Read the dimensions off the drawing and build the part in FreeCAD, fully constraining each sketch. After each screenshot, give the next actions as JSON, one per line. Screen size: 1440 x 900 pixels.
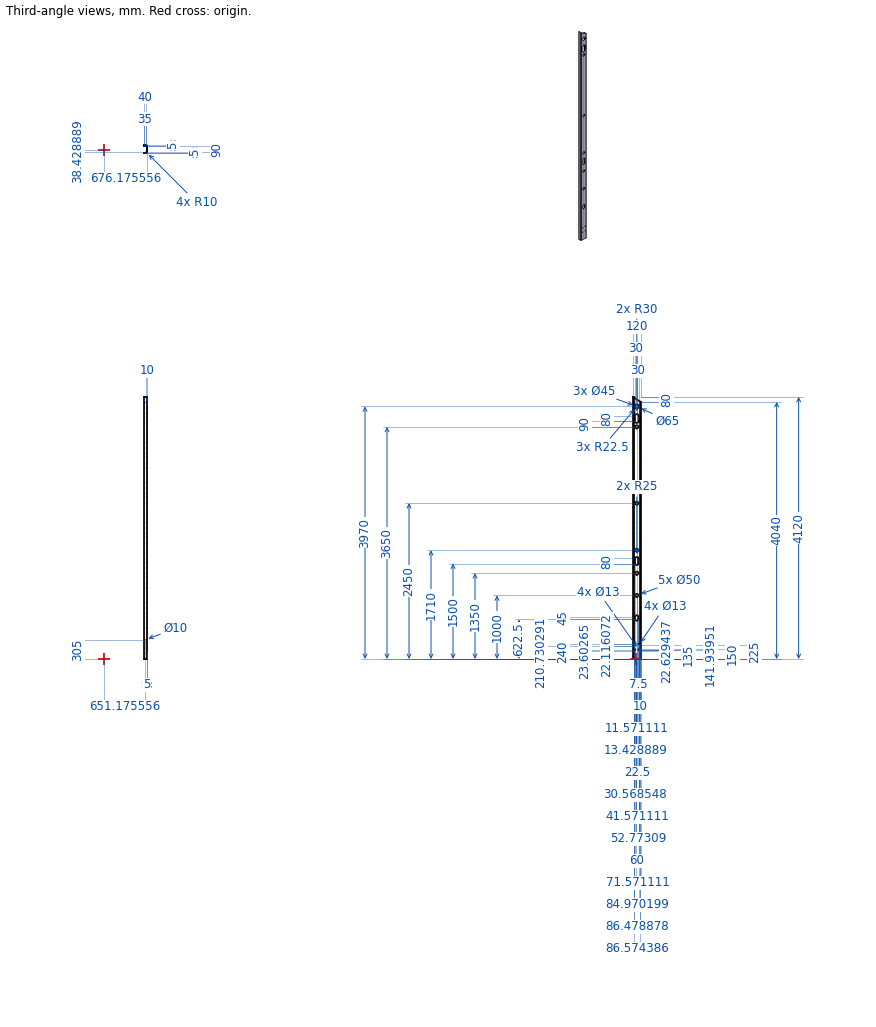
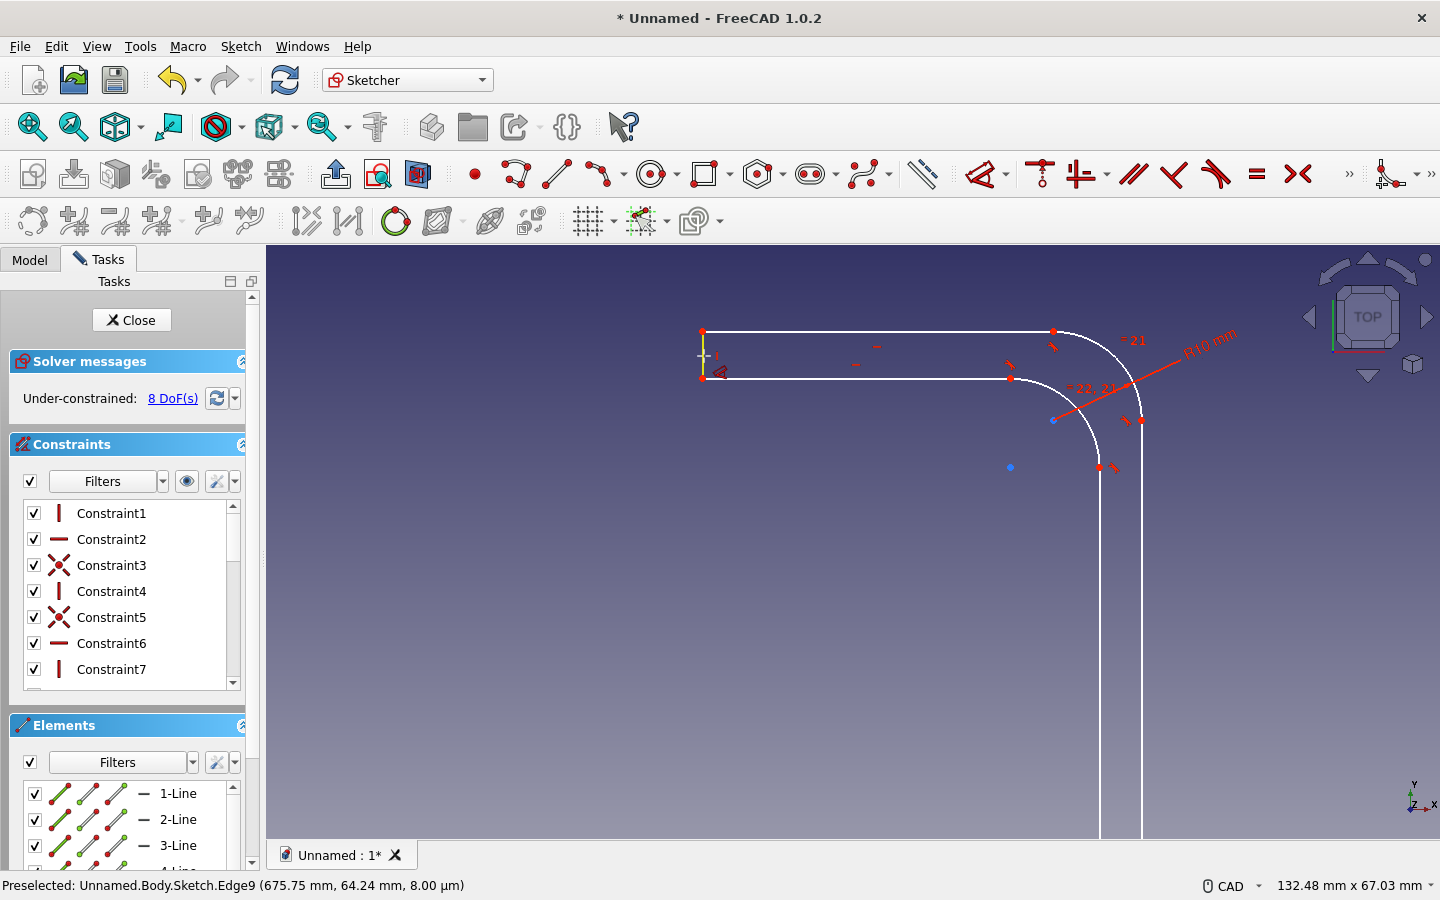
{"action": "left_click", "coordinate": [703, 355]}
{"action": "left_click", "coordinate": [669, 355]}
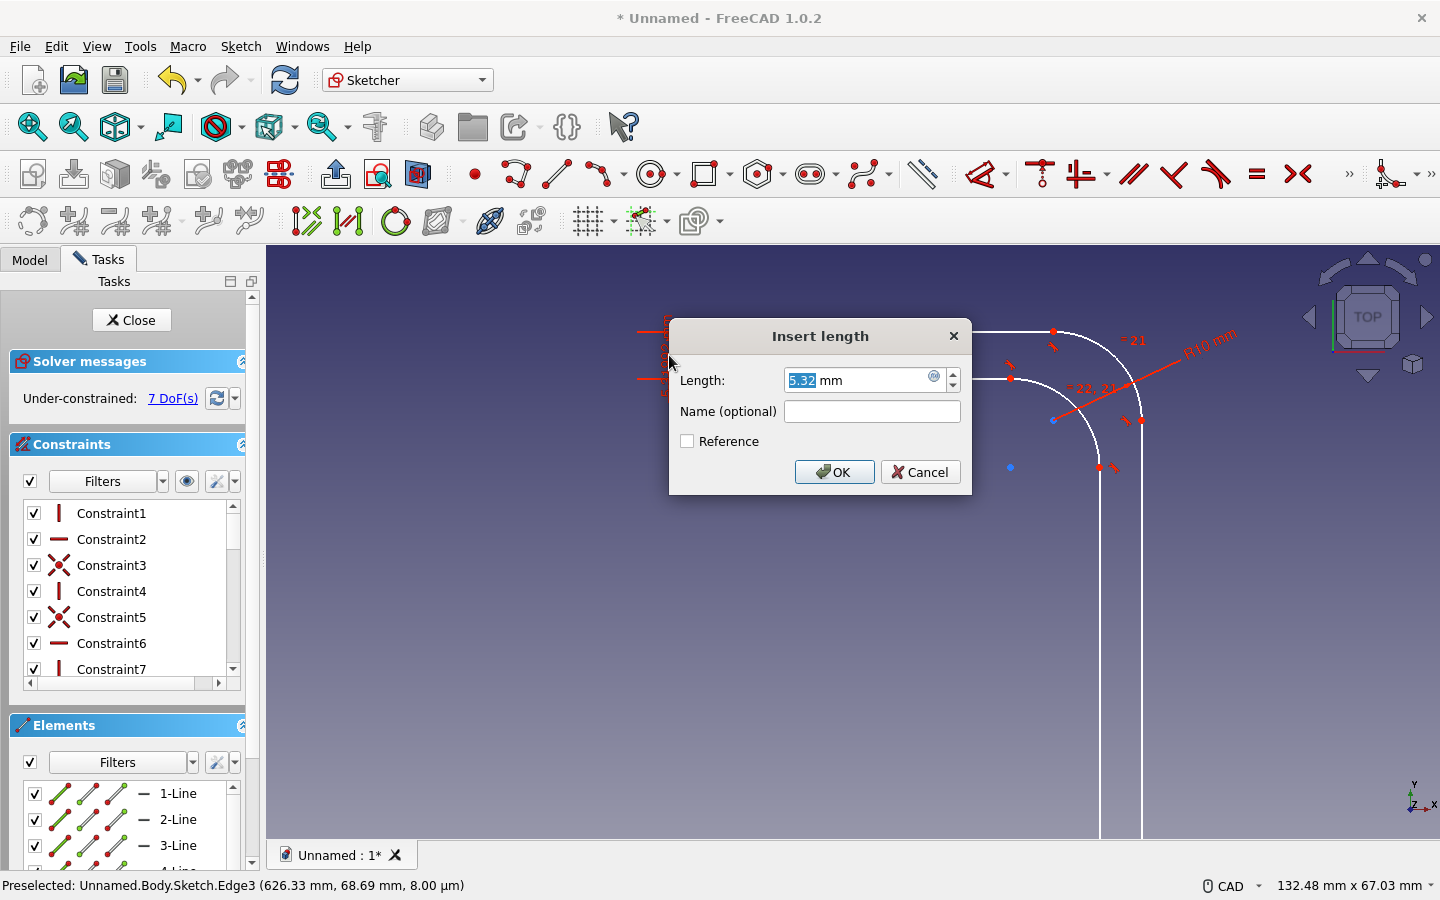
{"action": "type", "text": "5"}
{"action": "key", "text": "Return"}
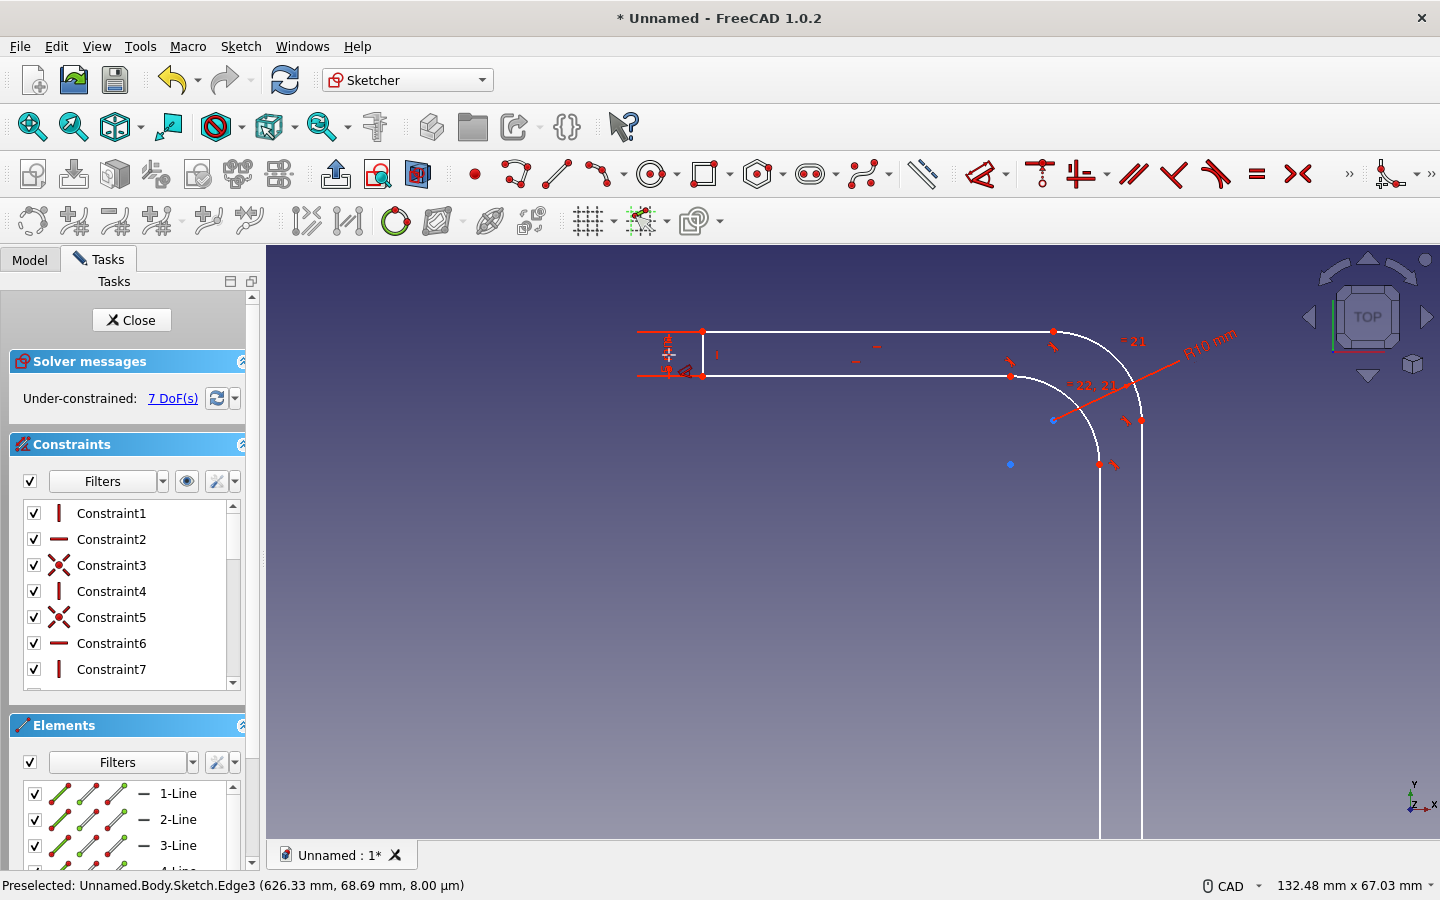
{"action": "scroll", "coordinate": [704, 356], "scroll_direction": "down", "scroll_amount": 5}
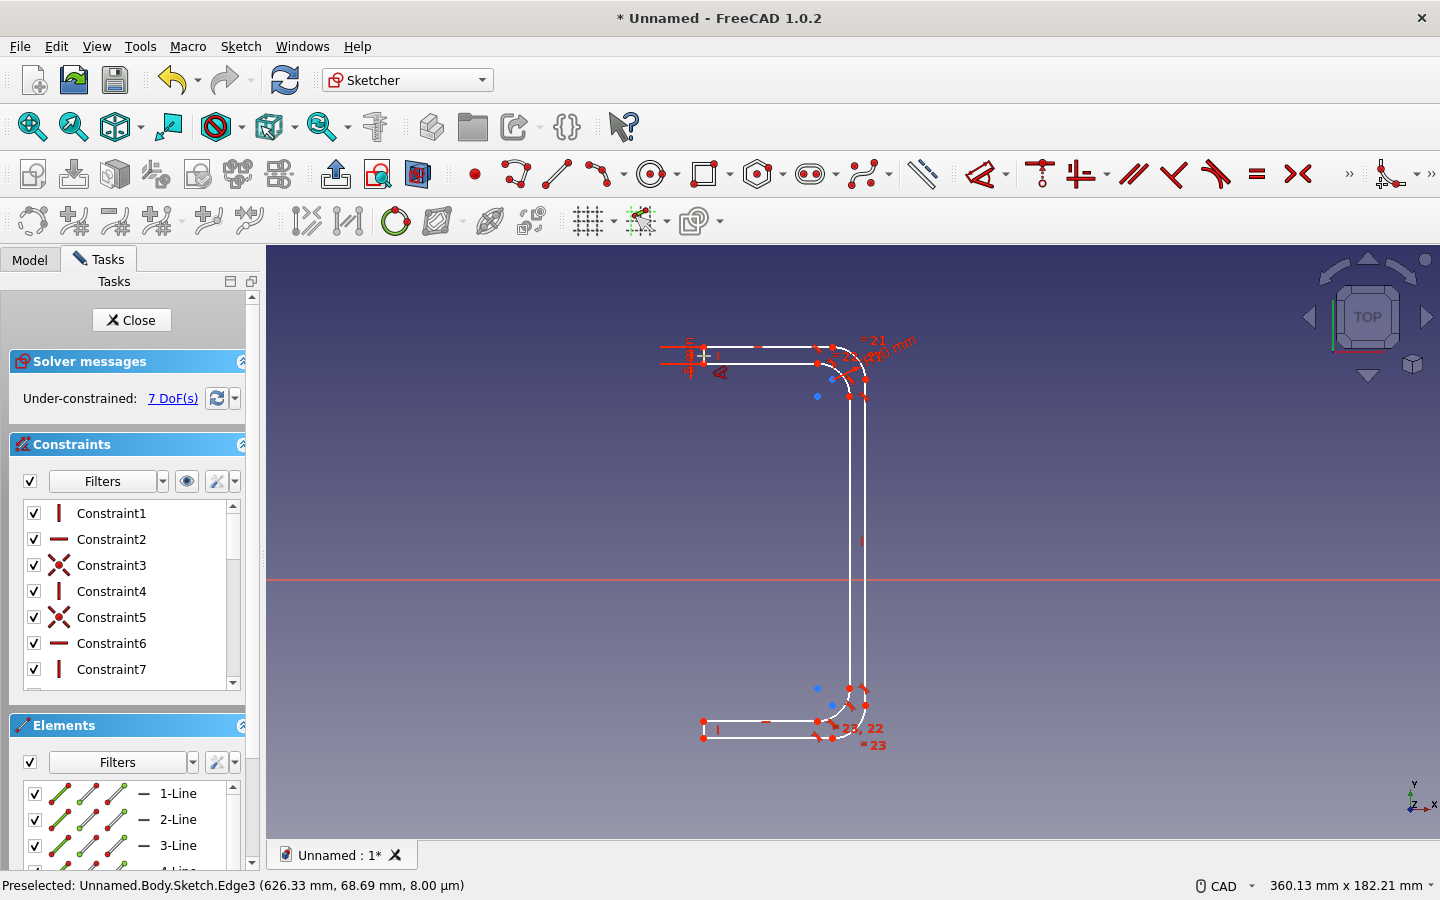
{"action": "scroll", "coordinate": [704, 726], "scroll_direction": "up", "scroll_amount": 5}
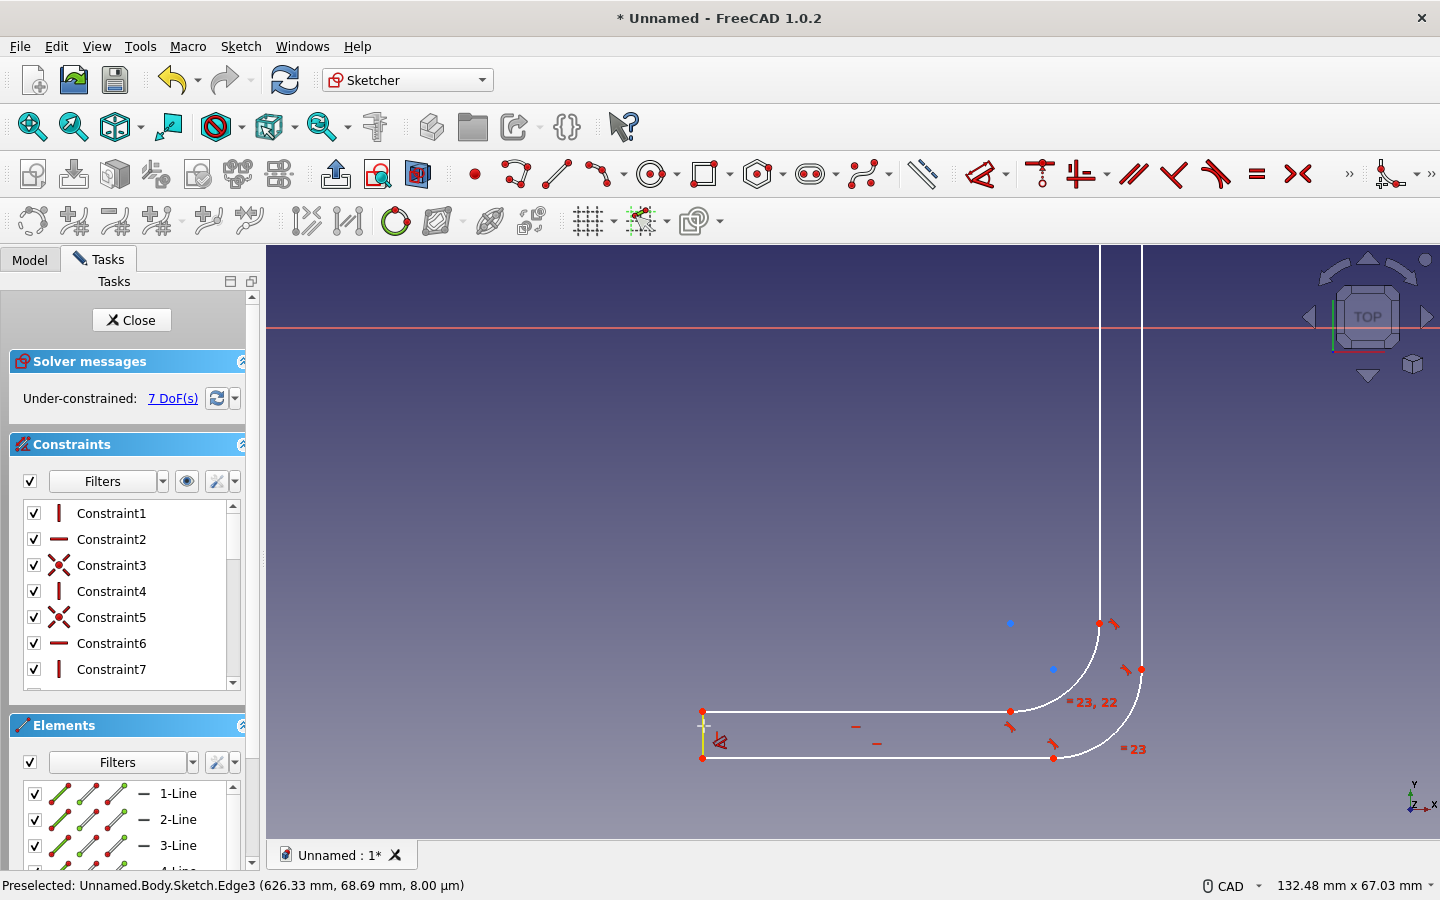
{"action": "left_click", "coordinate": [703, 726]}
{"action": "left_click", "coordinate": [669, 735]}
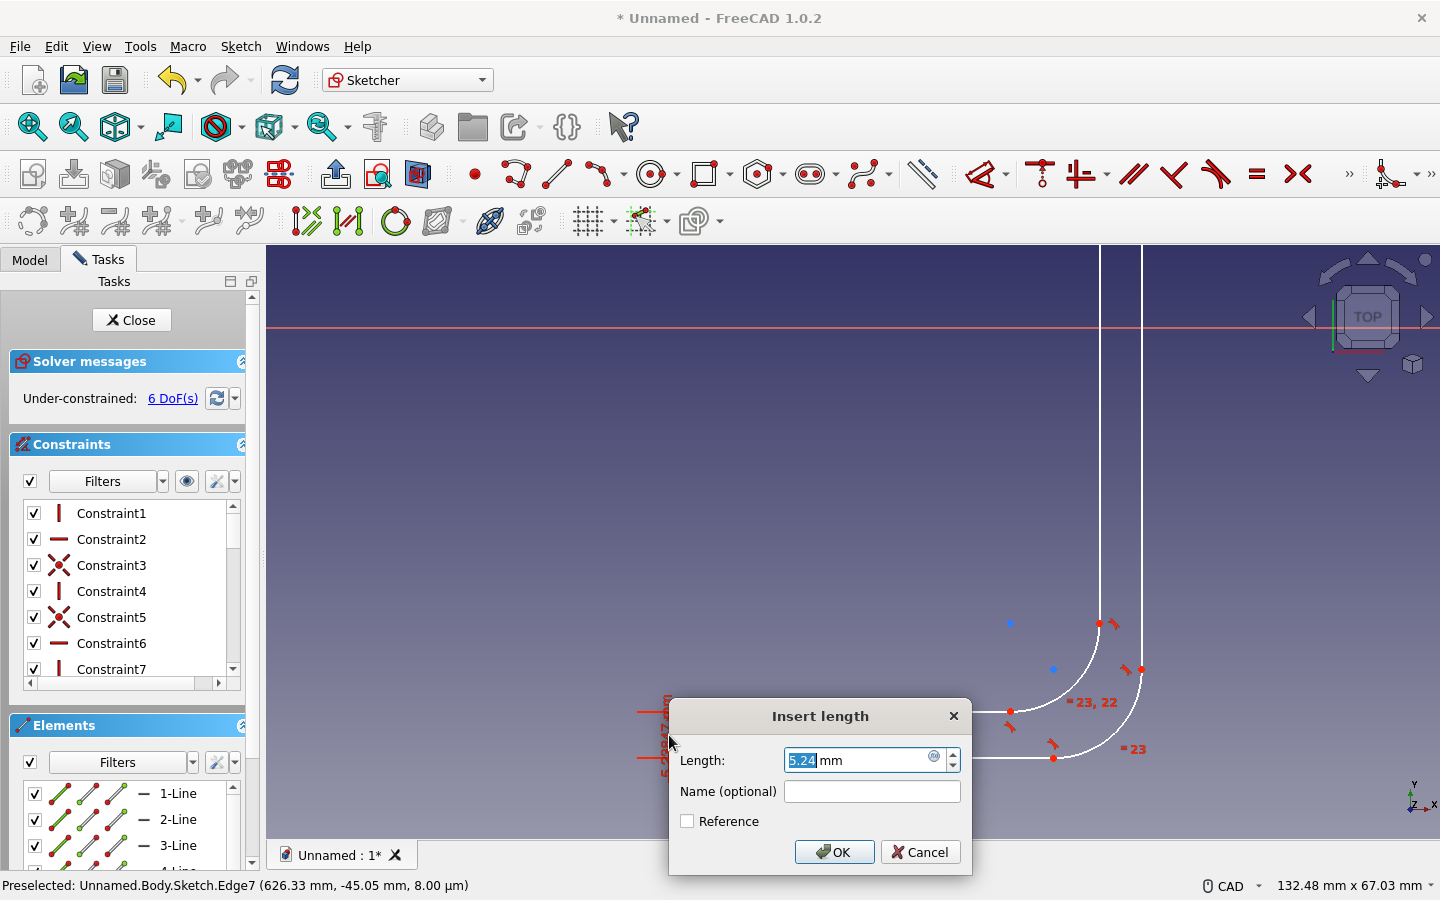
{"action": "type", "text": "5"}
{"action": "key", "text": "Return"}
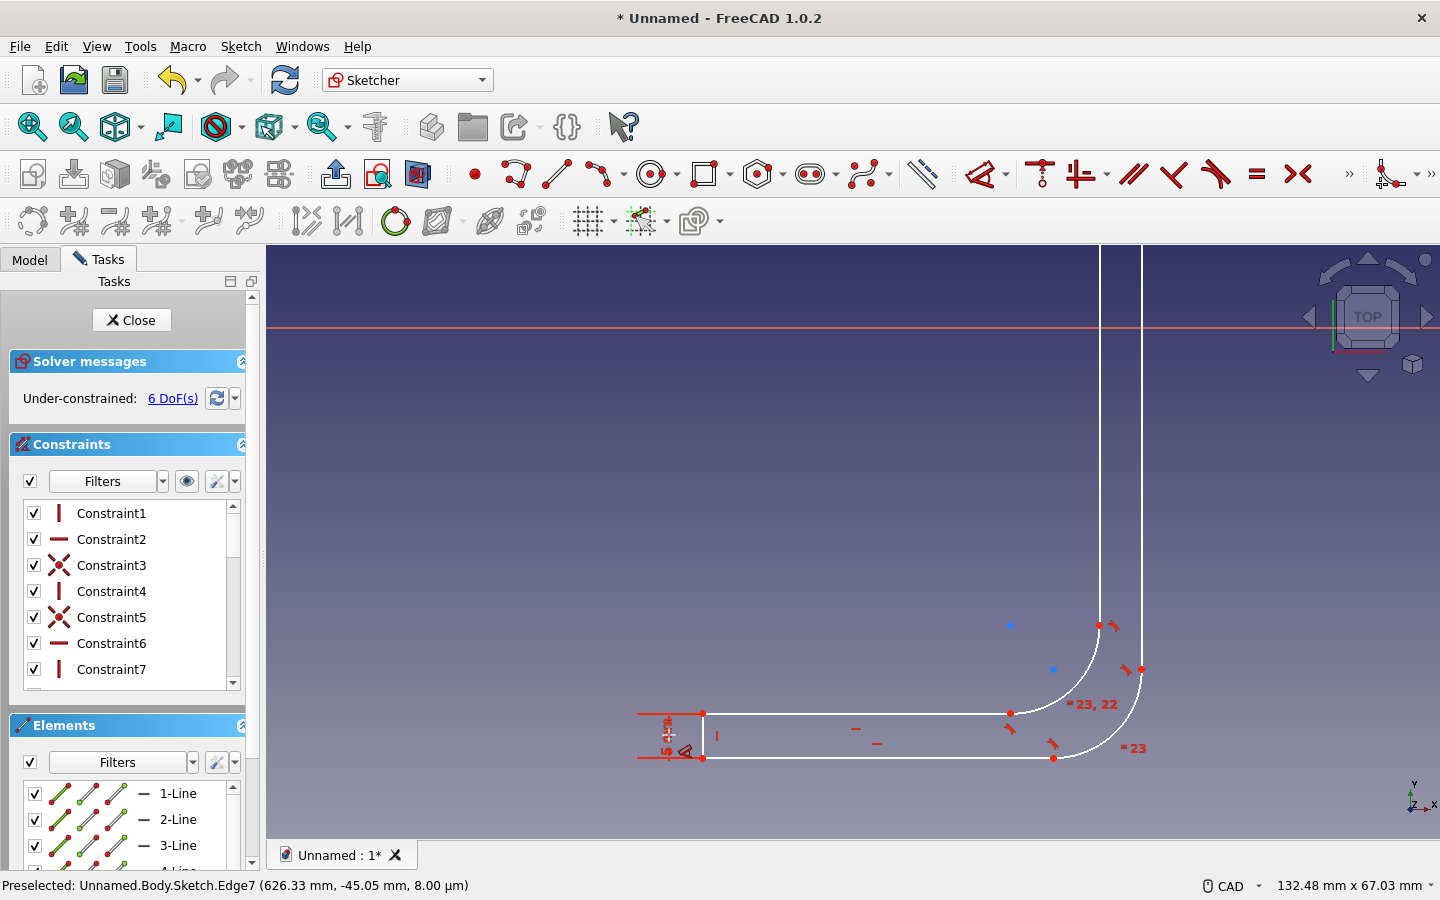
{"action": "scroll", "coordinate": [704, 726], "scroll_direction": "down", "scroll_amount": 5}